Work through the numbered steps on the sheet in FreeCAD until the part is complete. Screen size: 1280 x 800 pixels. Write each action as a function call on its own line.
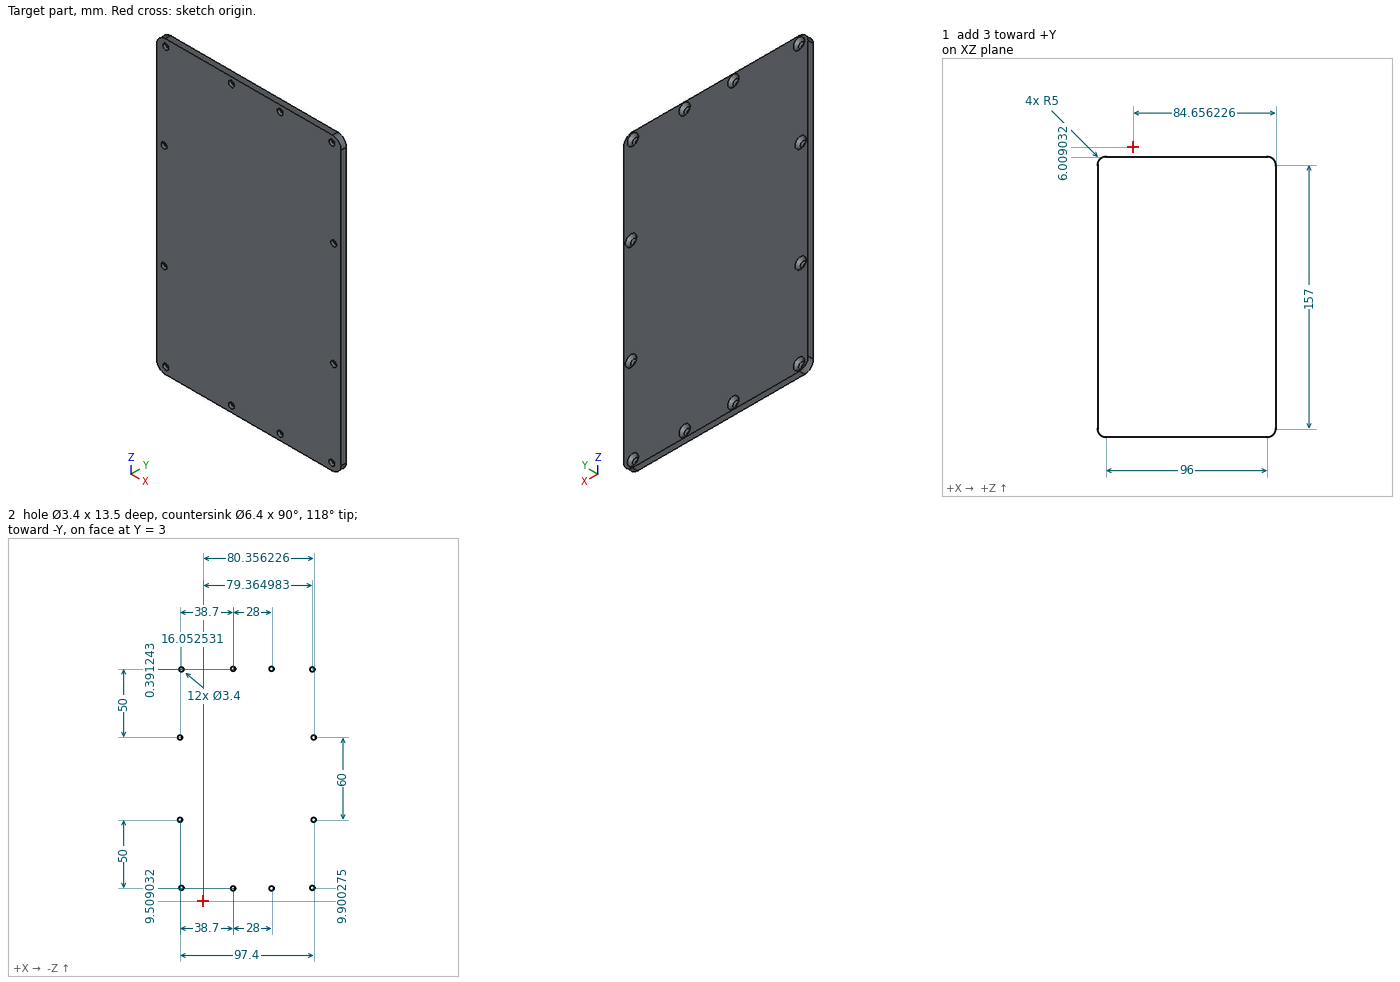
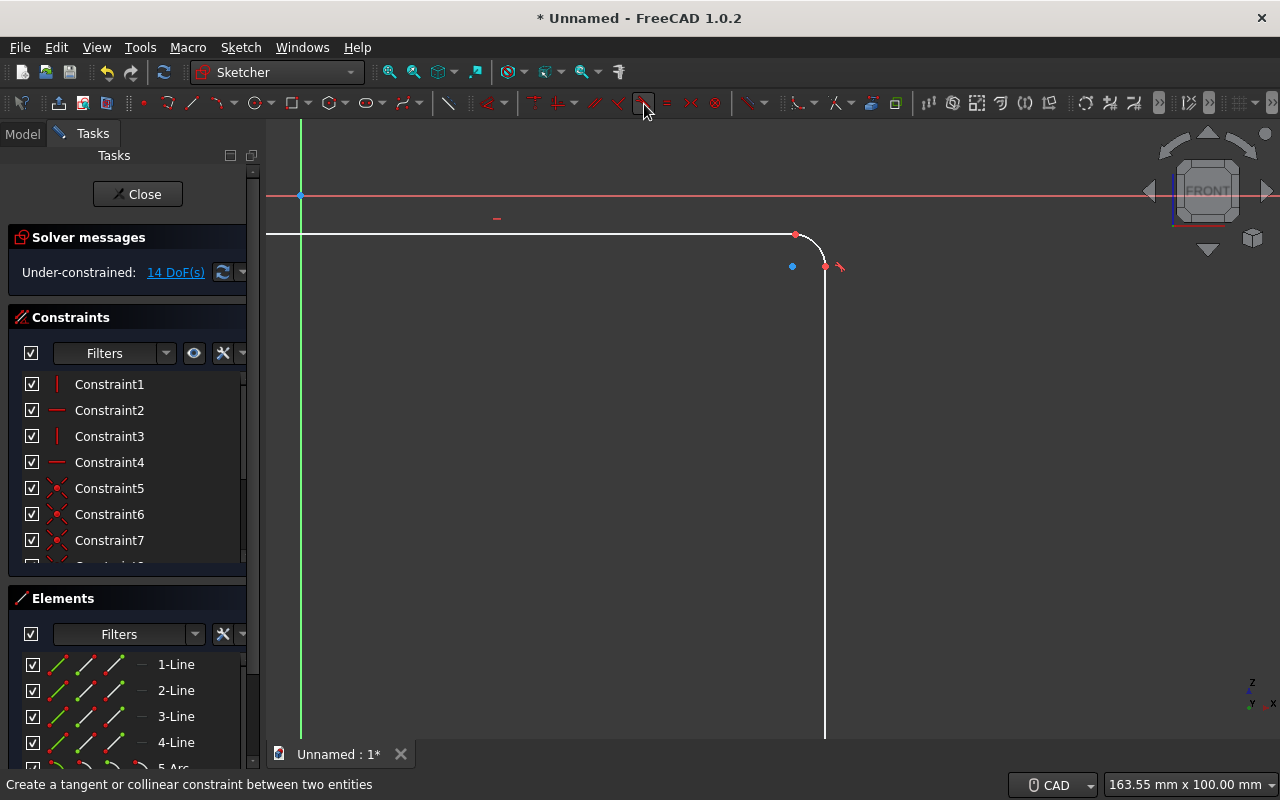
scroll(825, 253, down, 5)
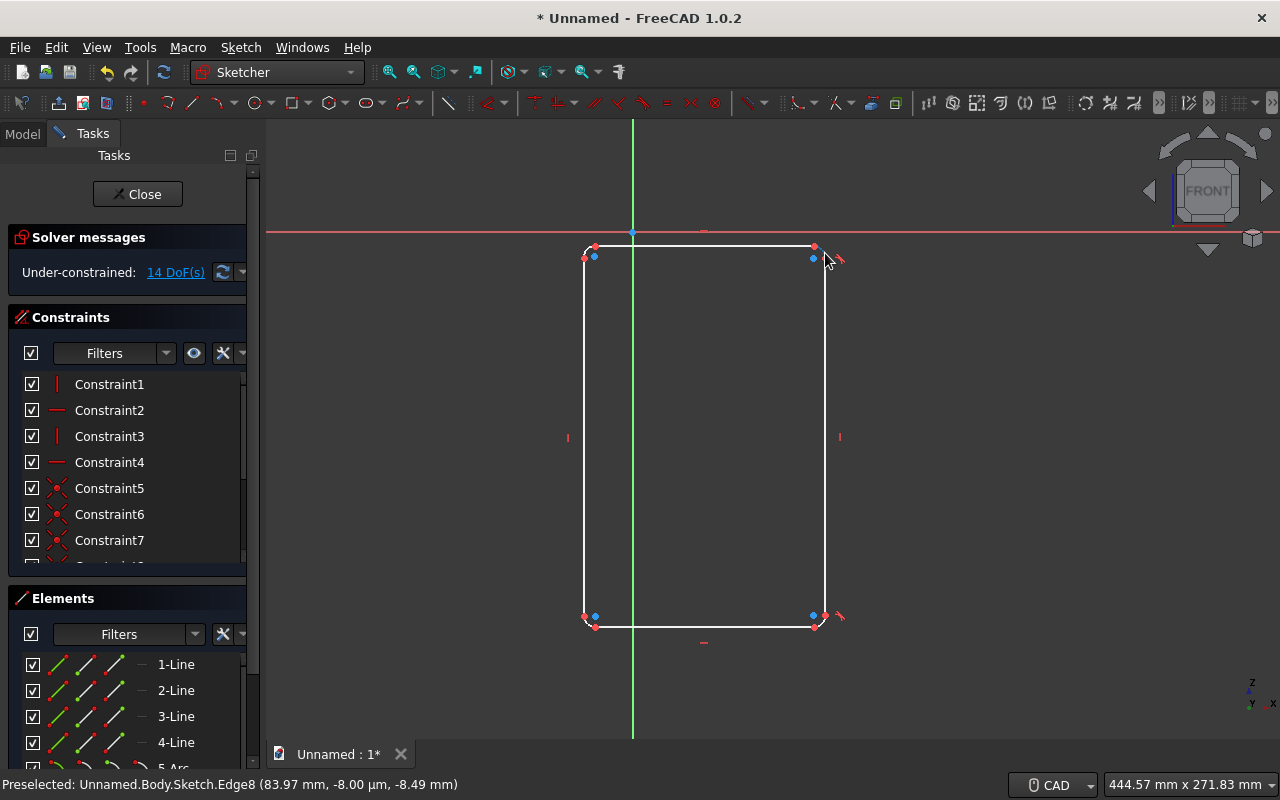
click(749, 627)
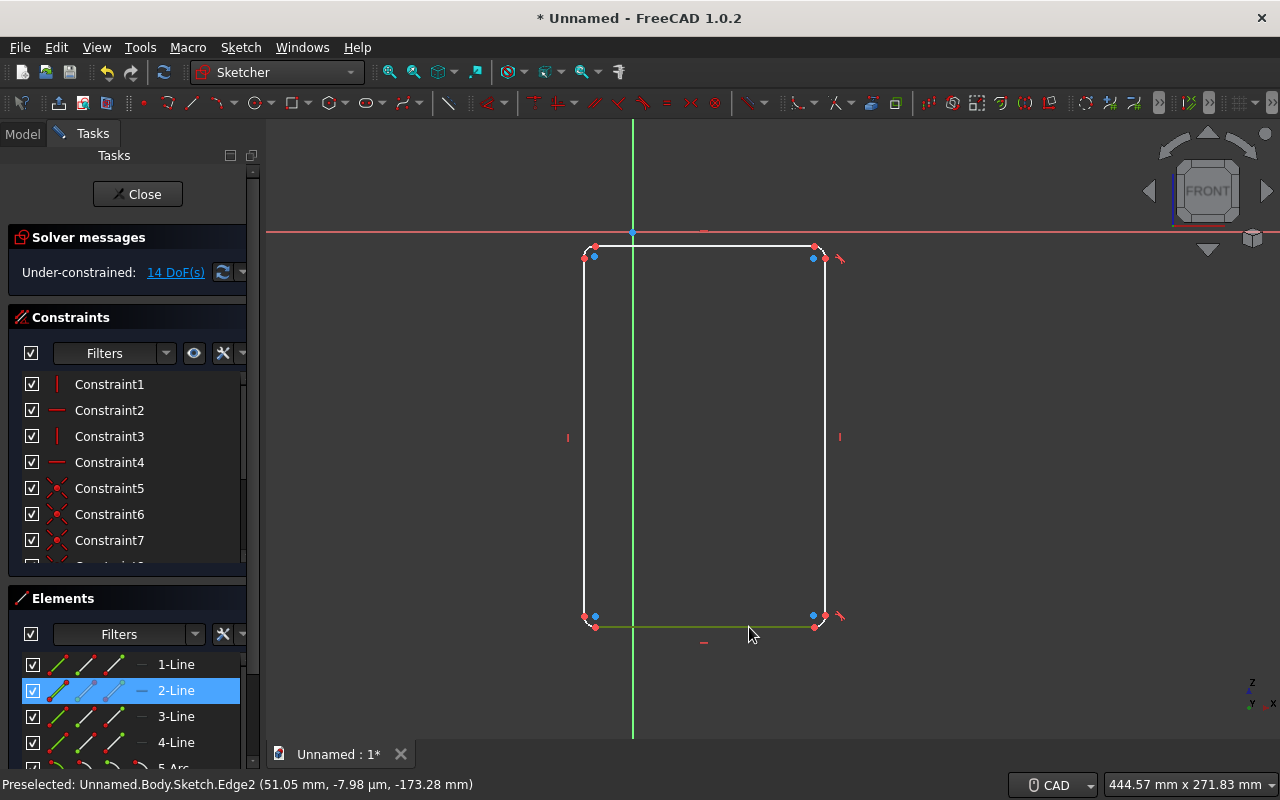
scroll(822, 624, up, 3)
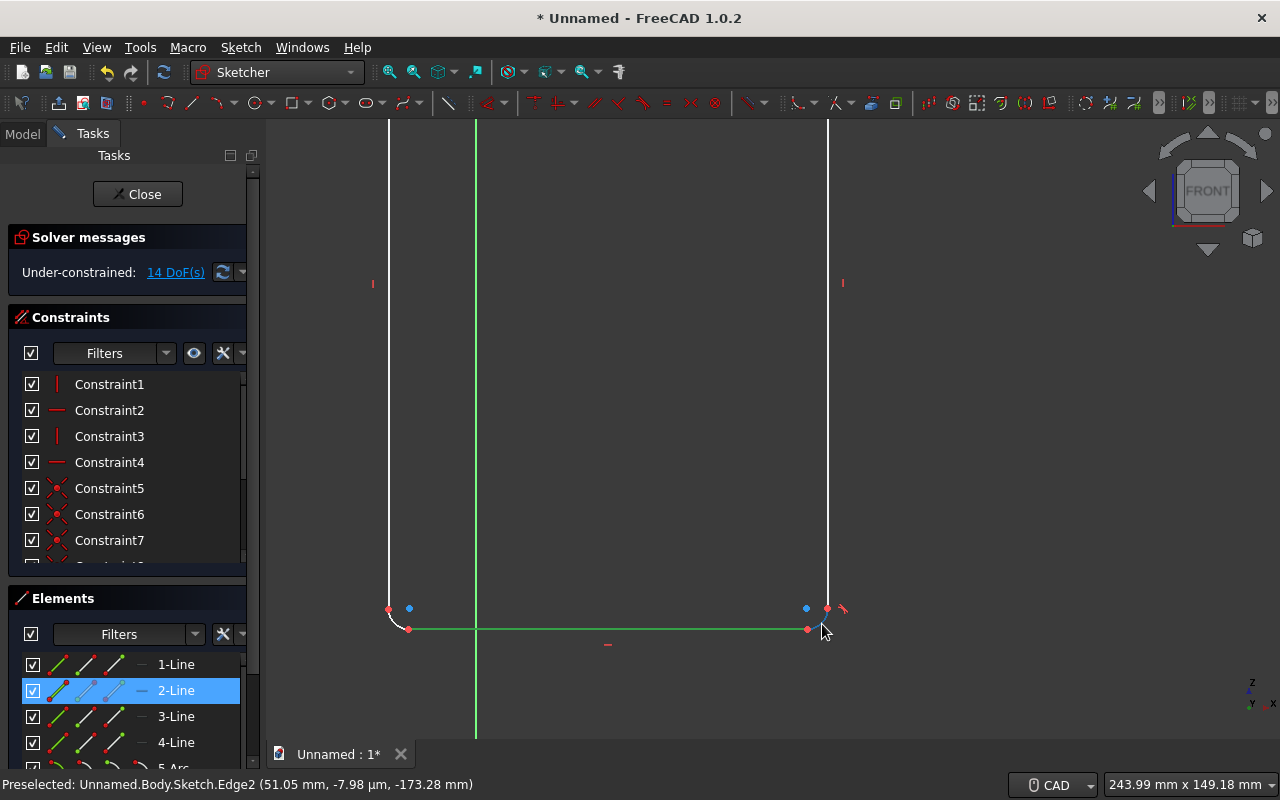
click(822, 623)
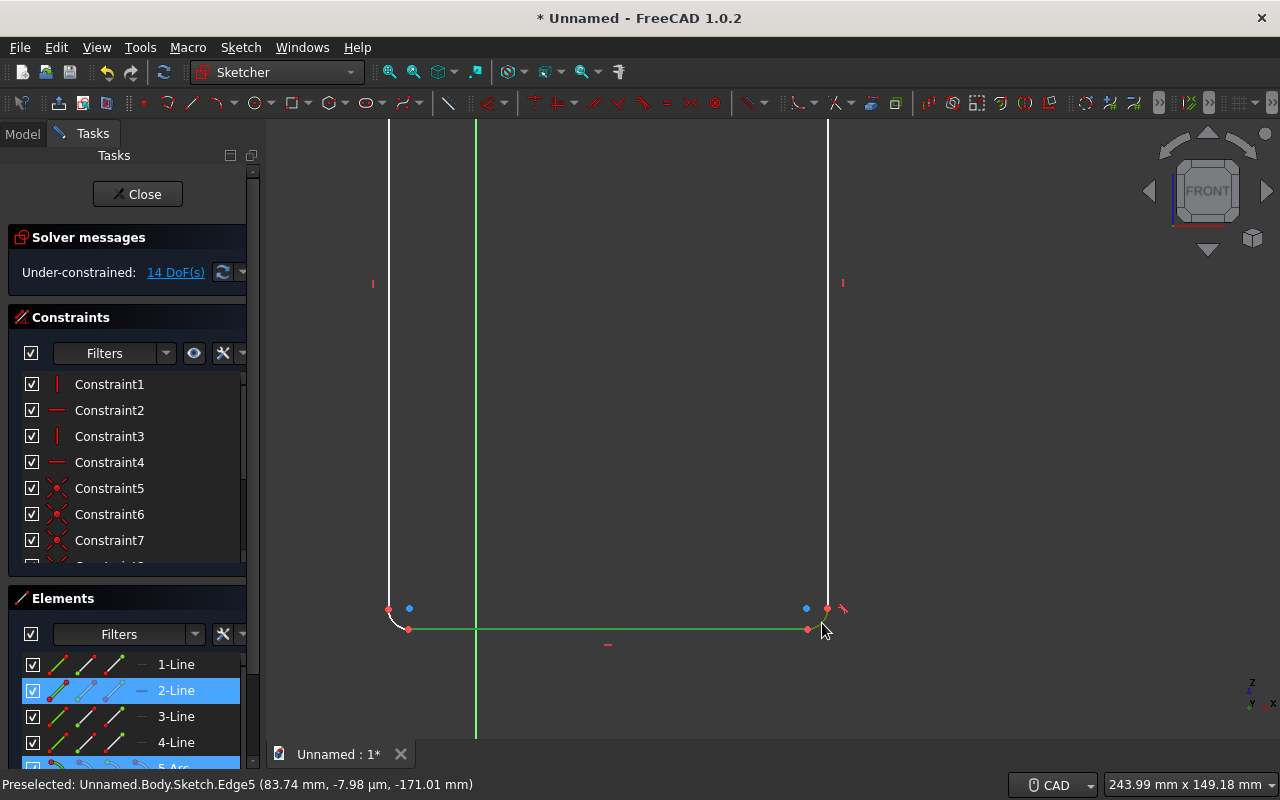
click(644, 104)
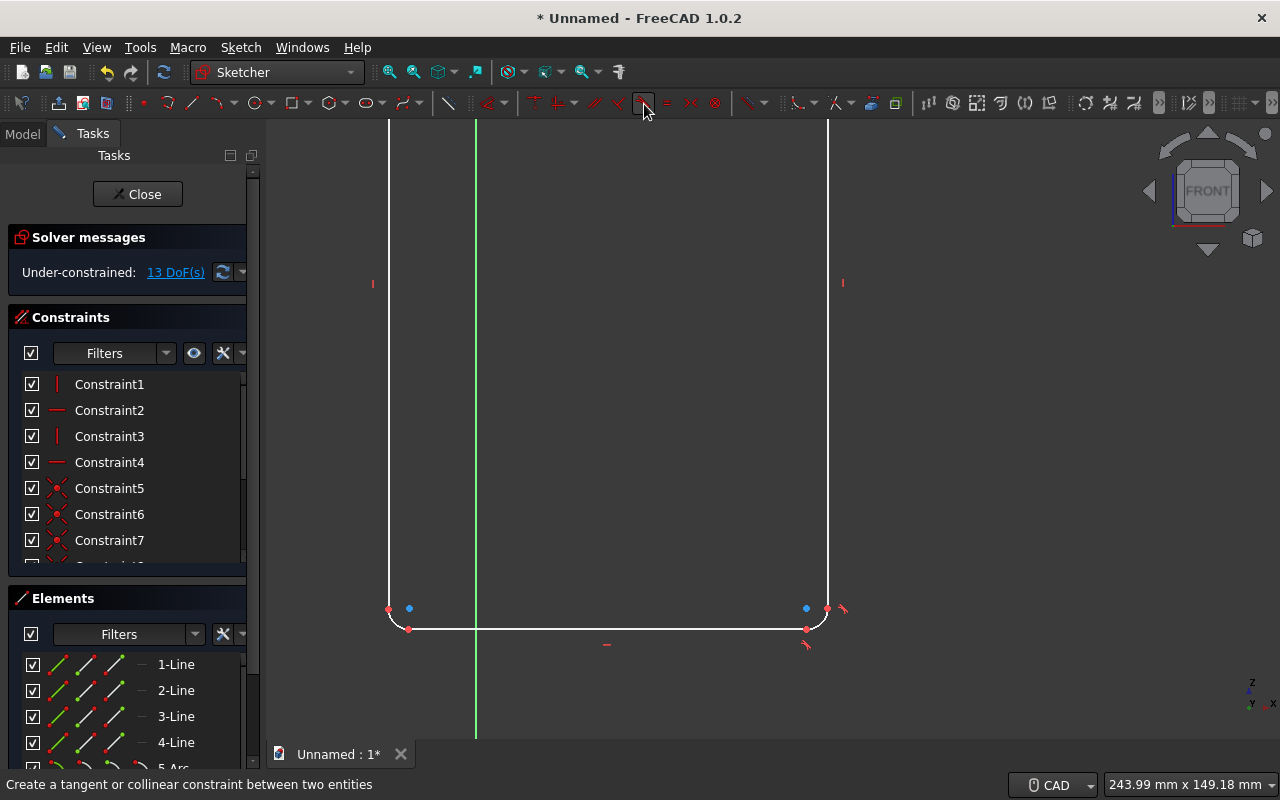
click(687, 629)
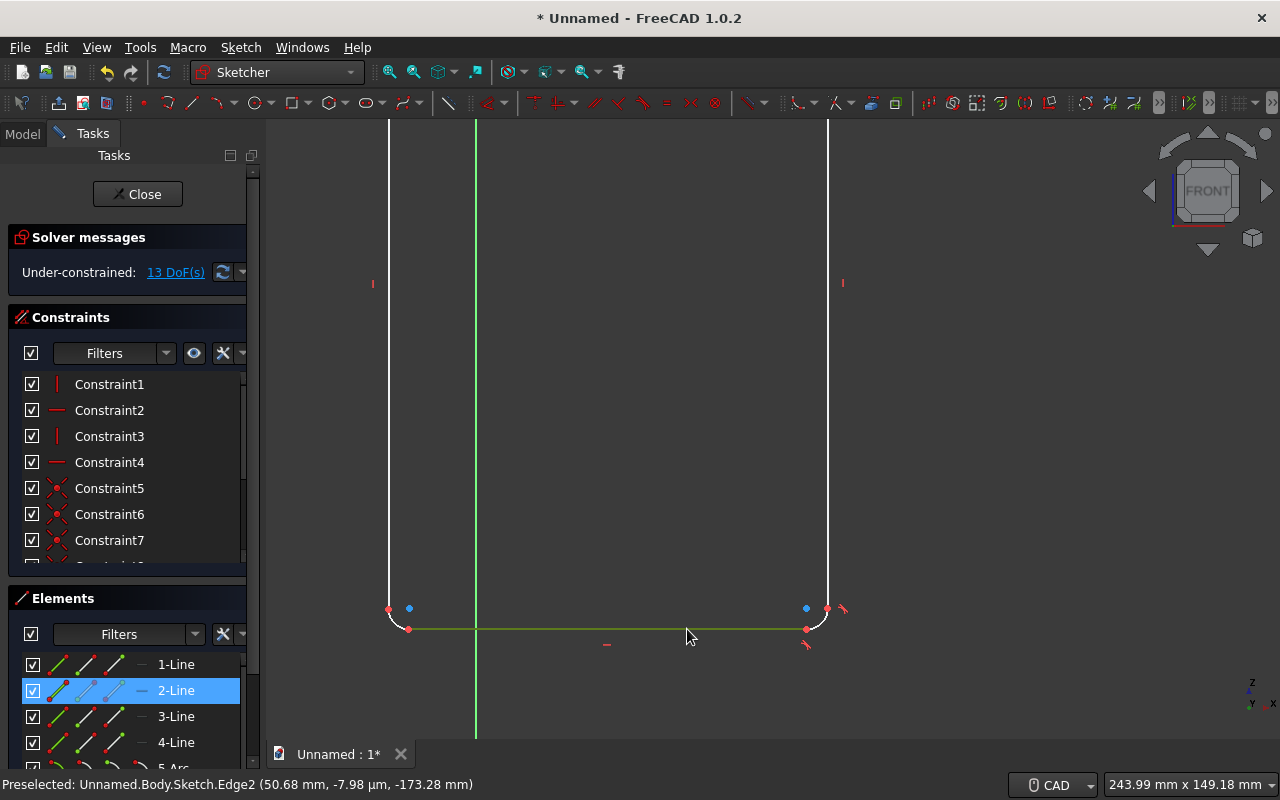
scroll(391, 618, up, 2)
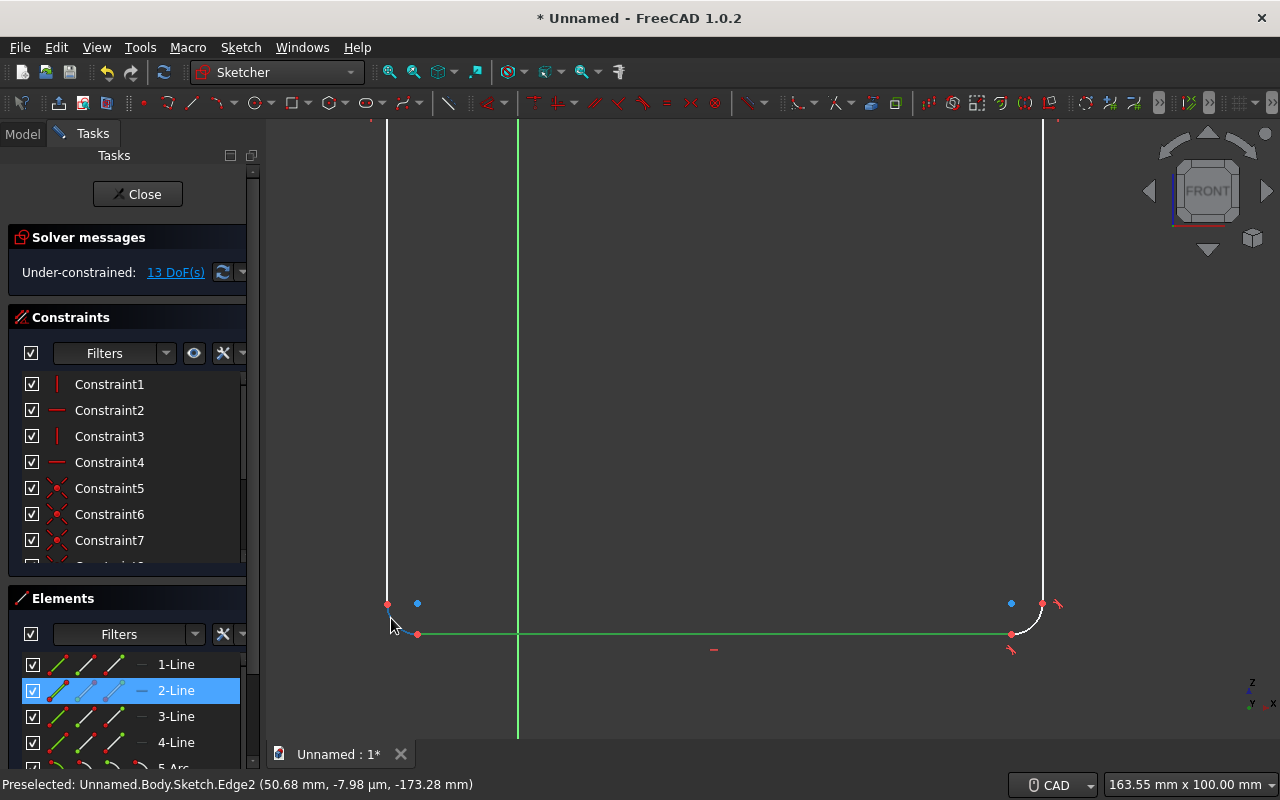
click(391, 618)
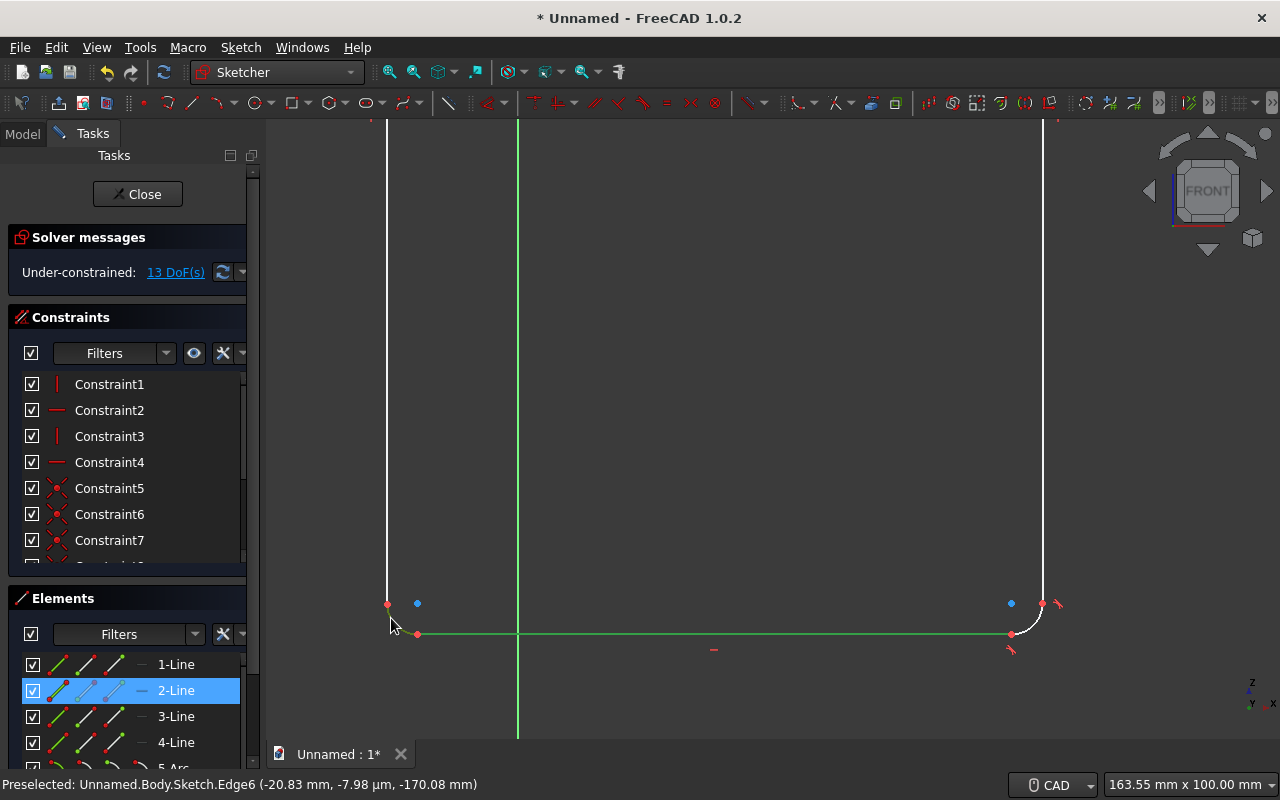
click(644, 104)